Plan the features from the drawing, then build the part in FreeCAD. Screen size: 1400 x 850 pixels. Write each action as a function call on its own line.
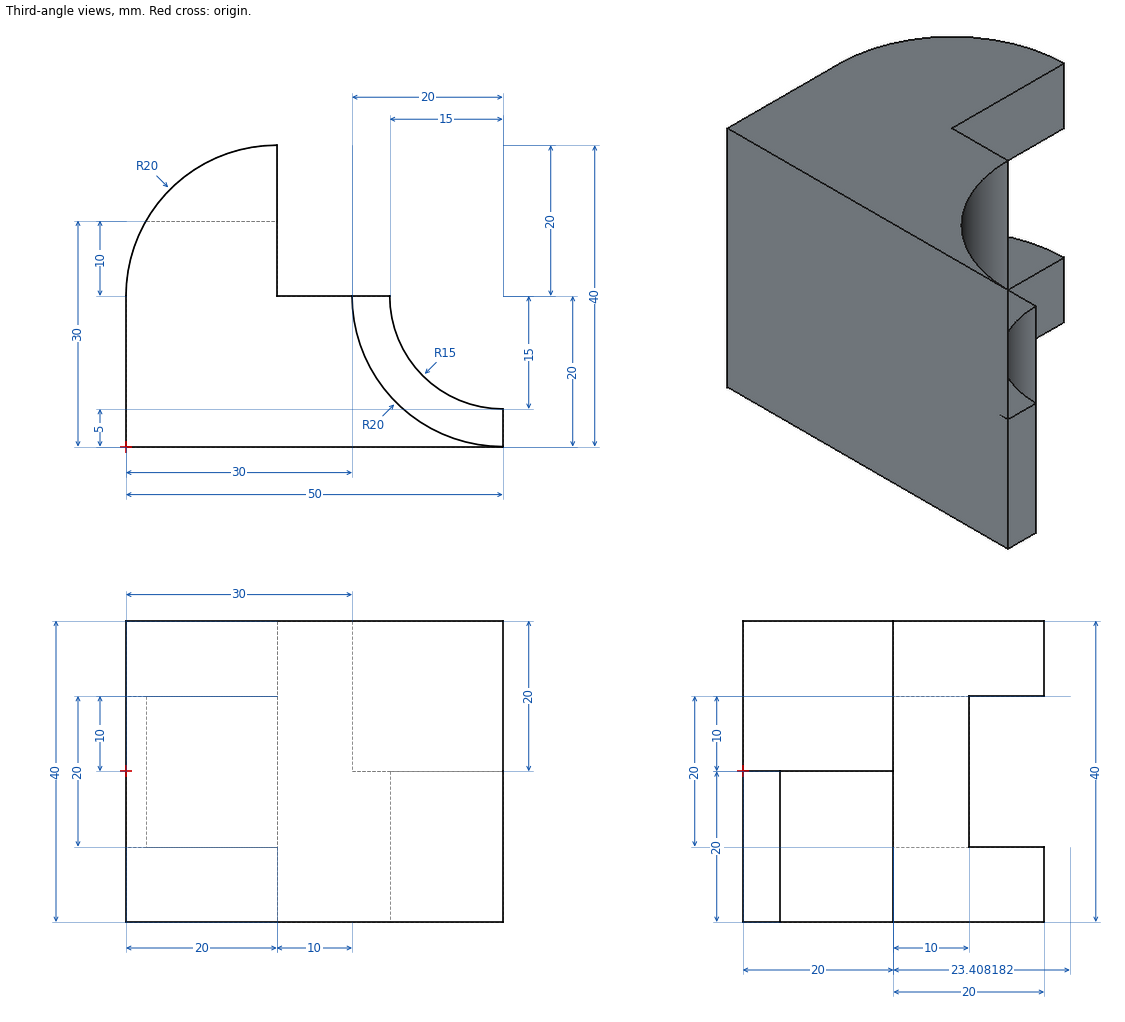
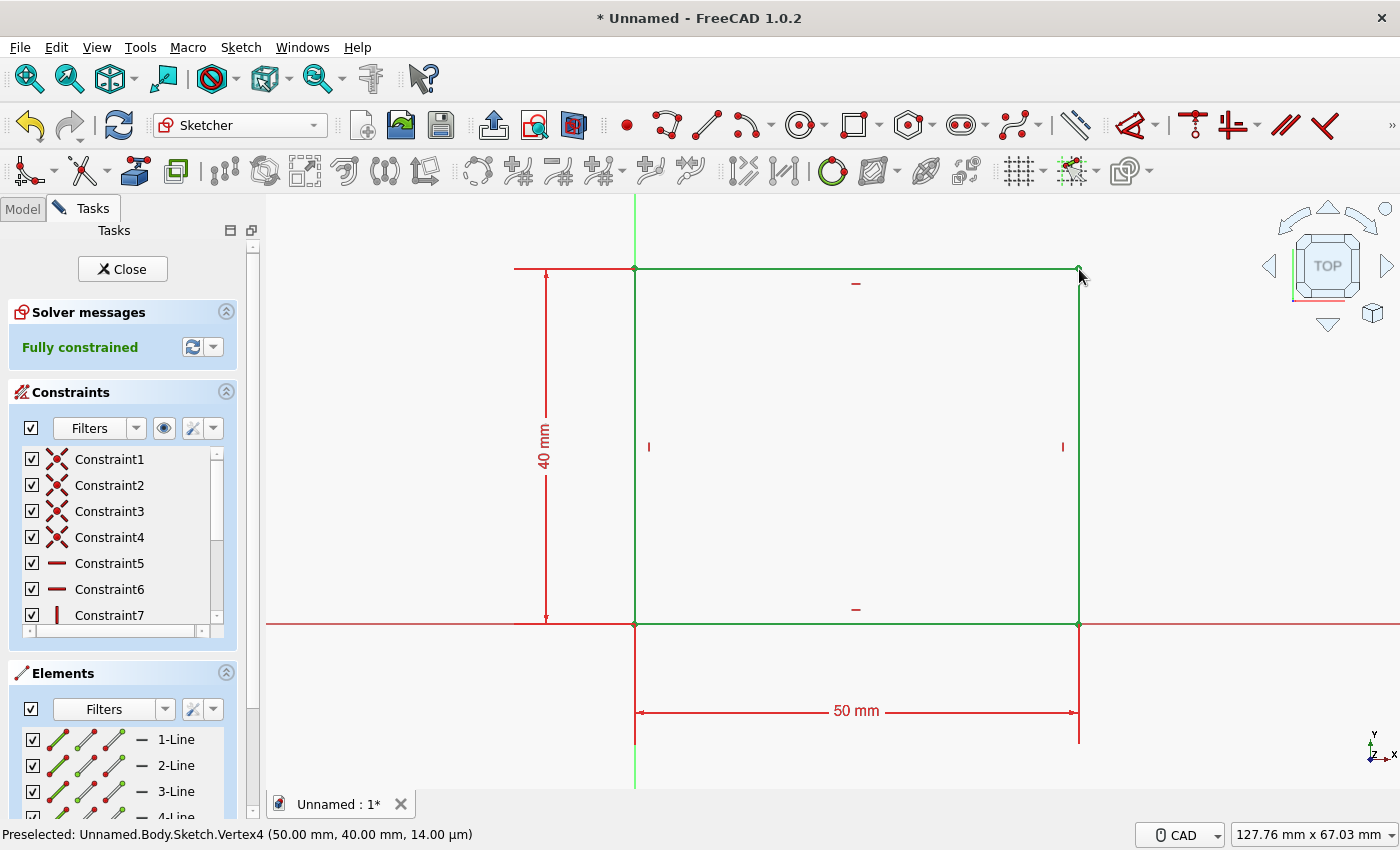
click(123, 269)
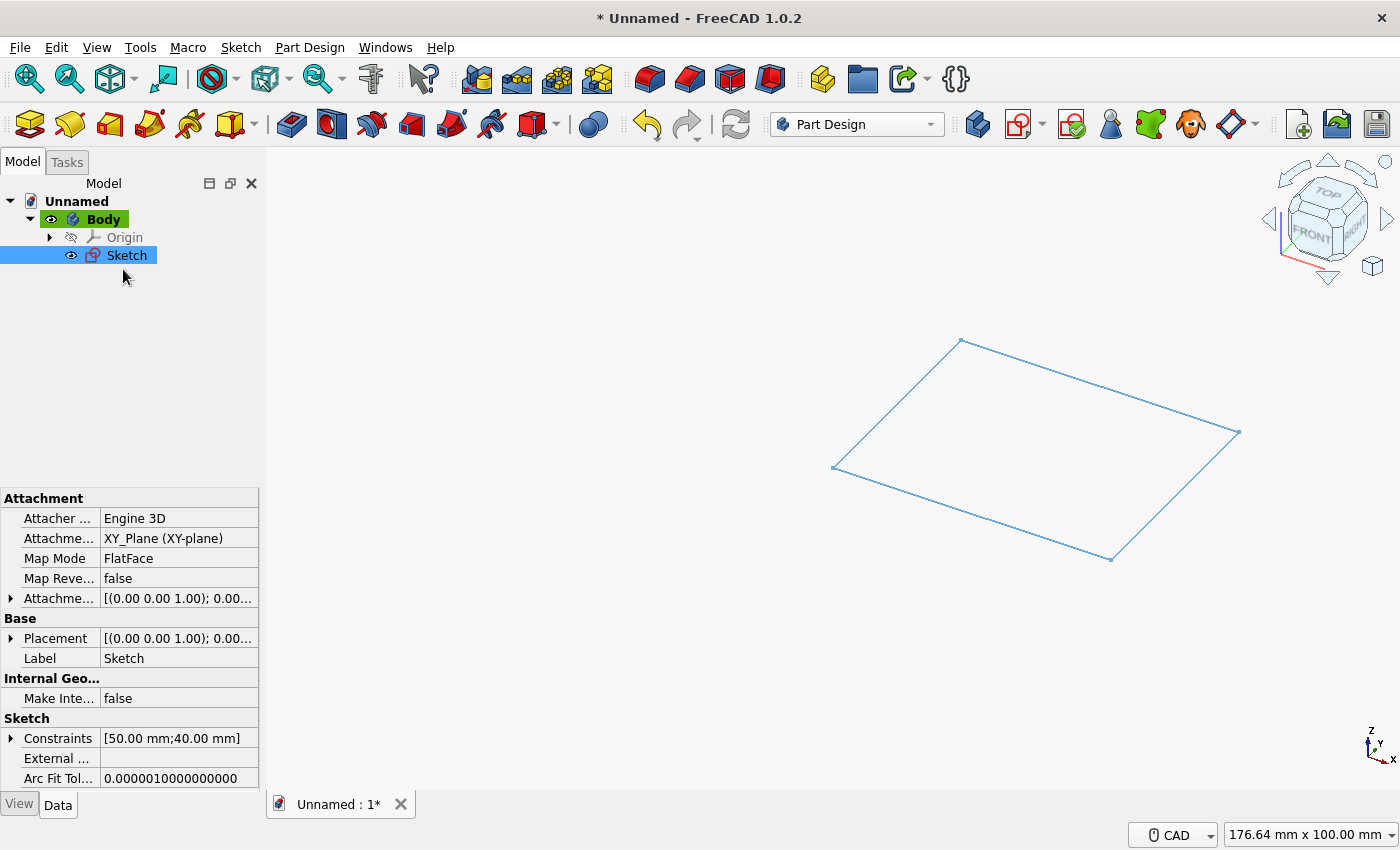
click(30, 124)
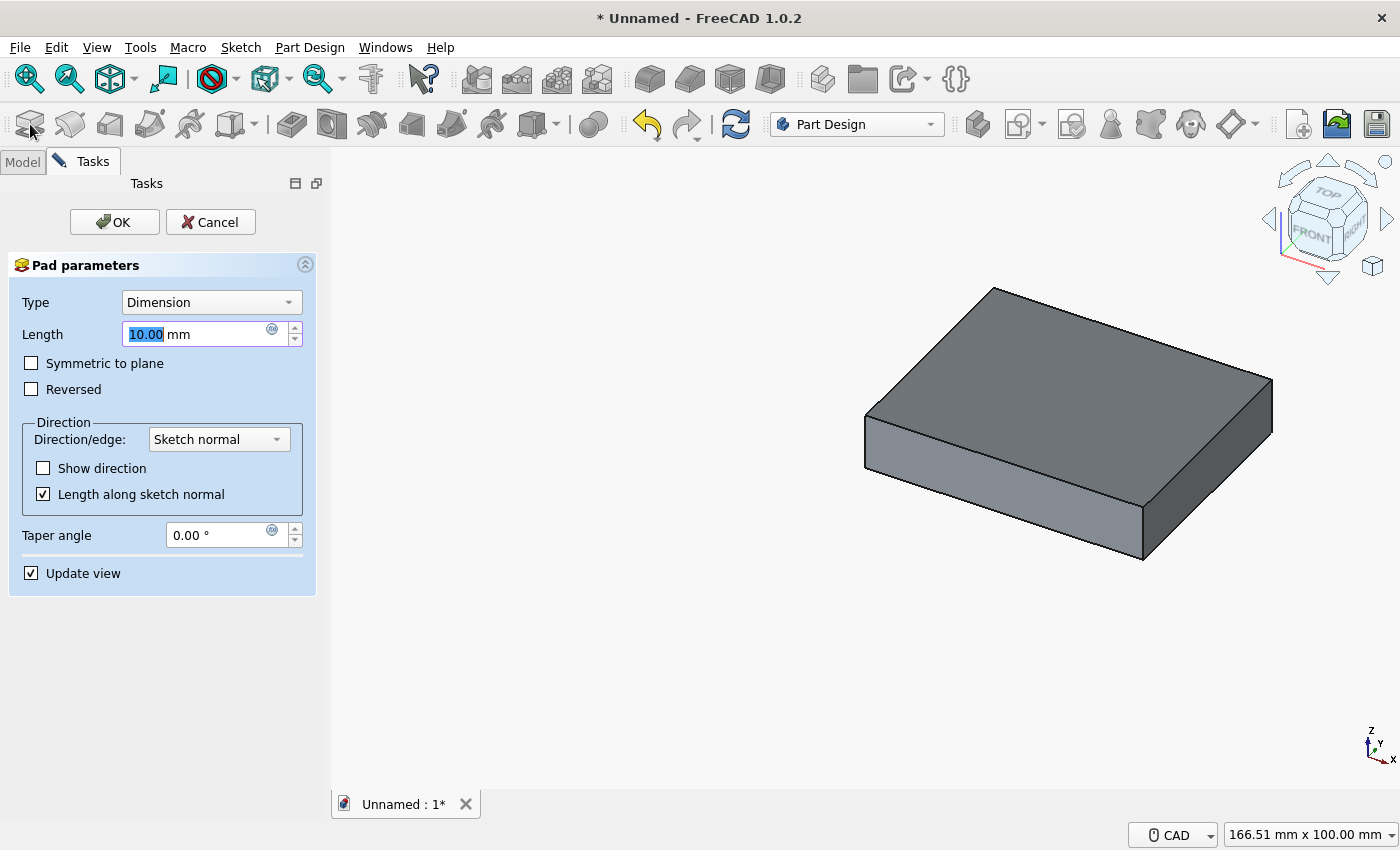
text(40)
key(Tab)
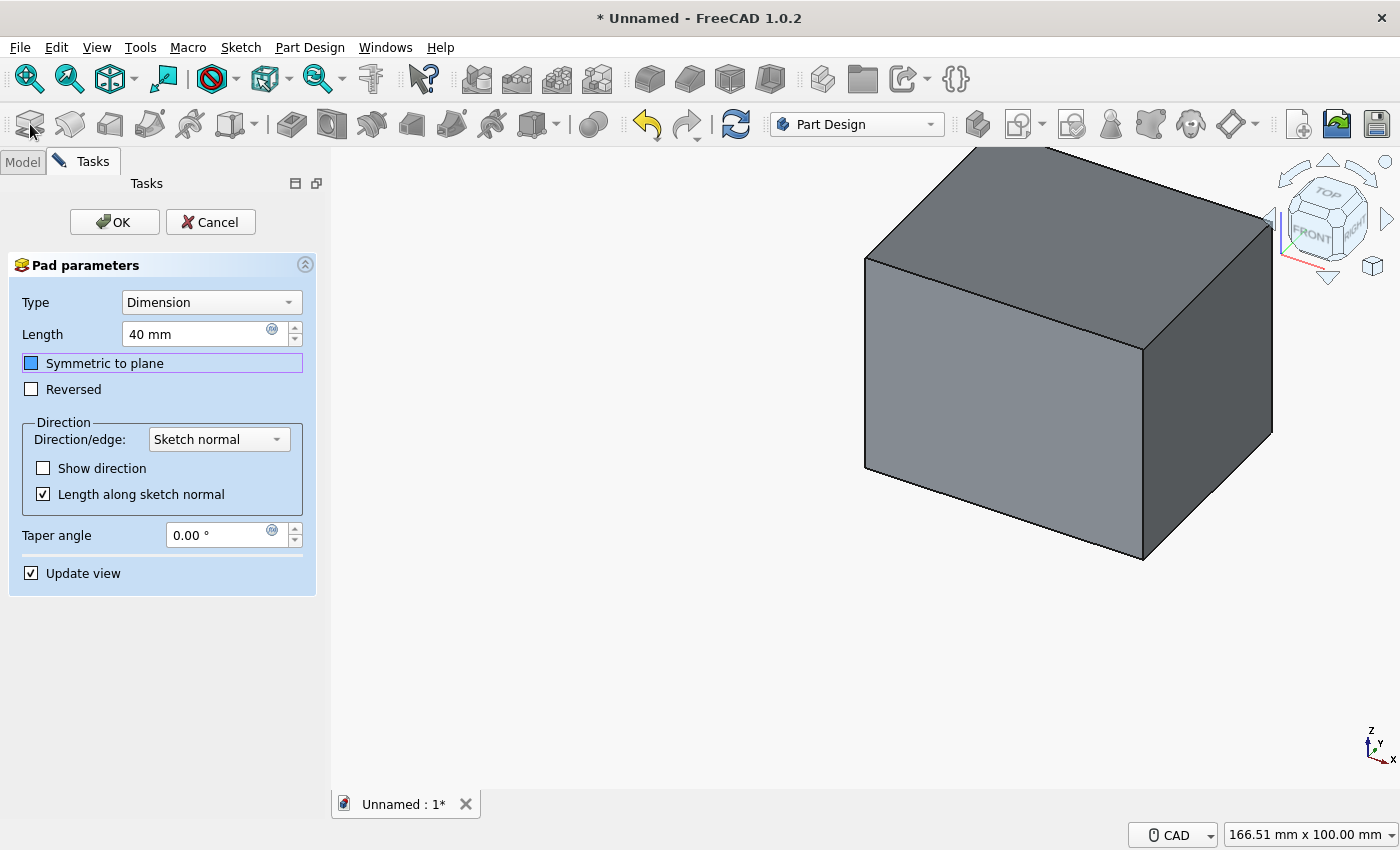
click(30, 363)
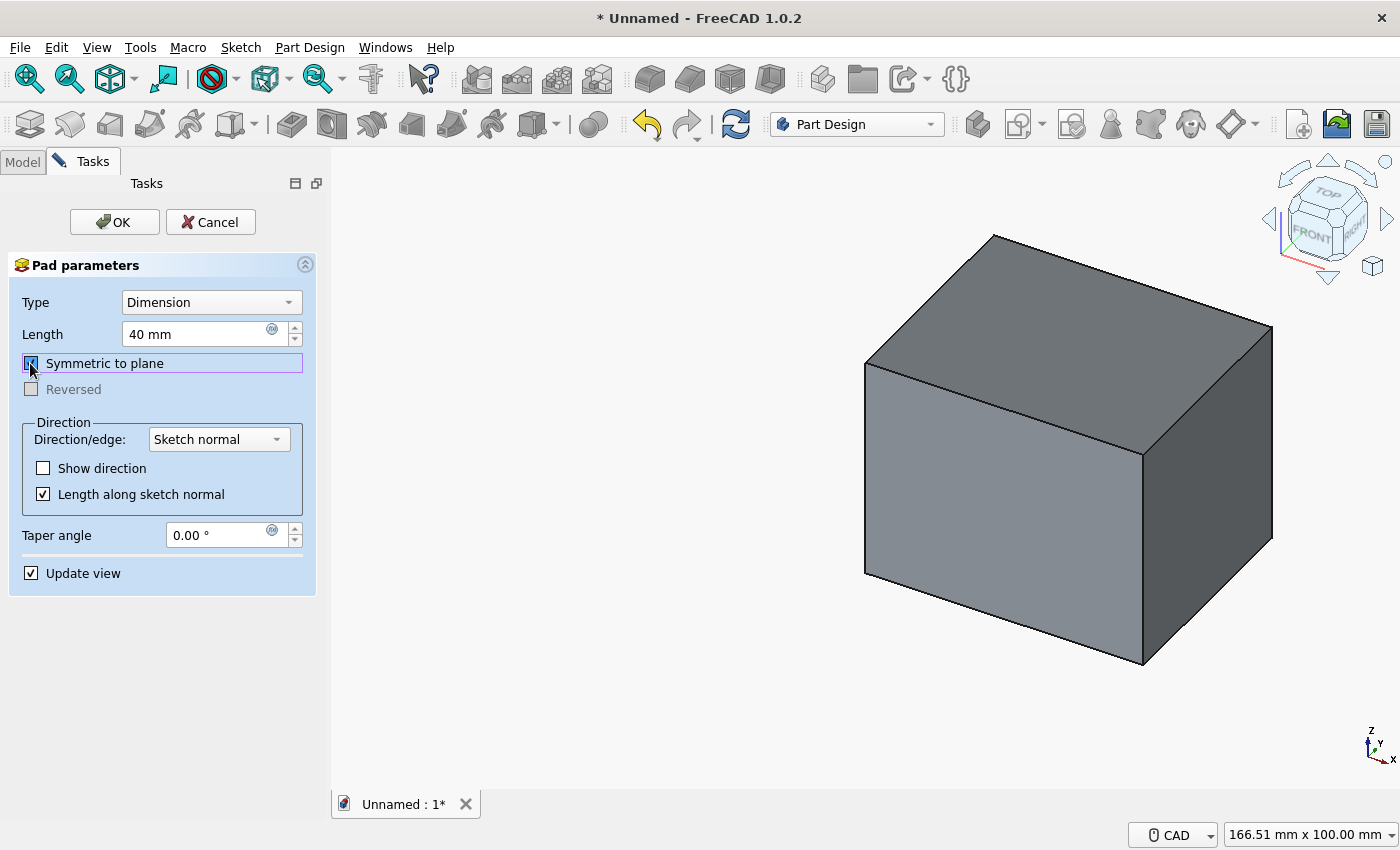
click(115, 222)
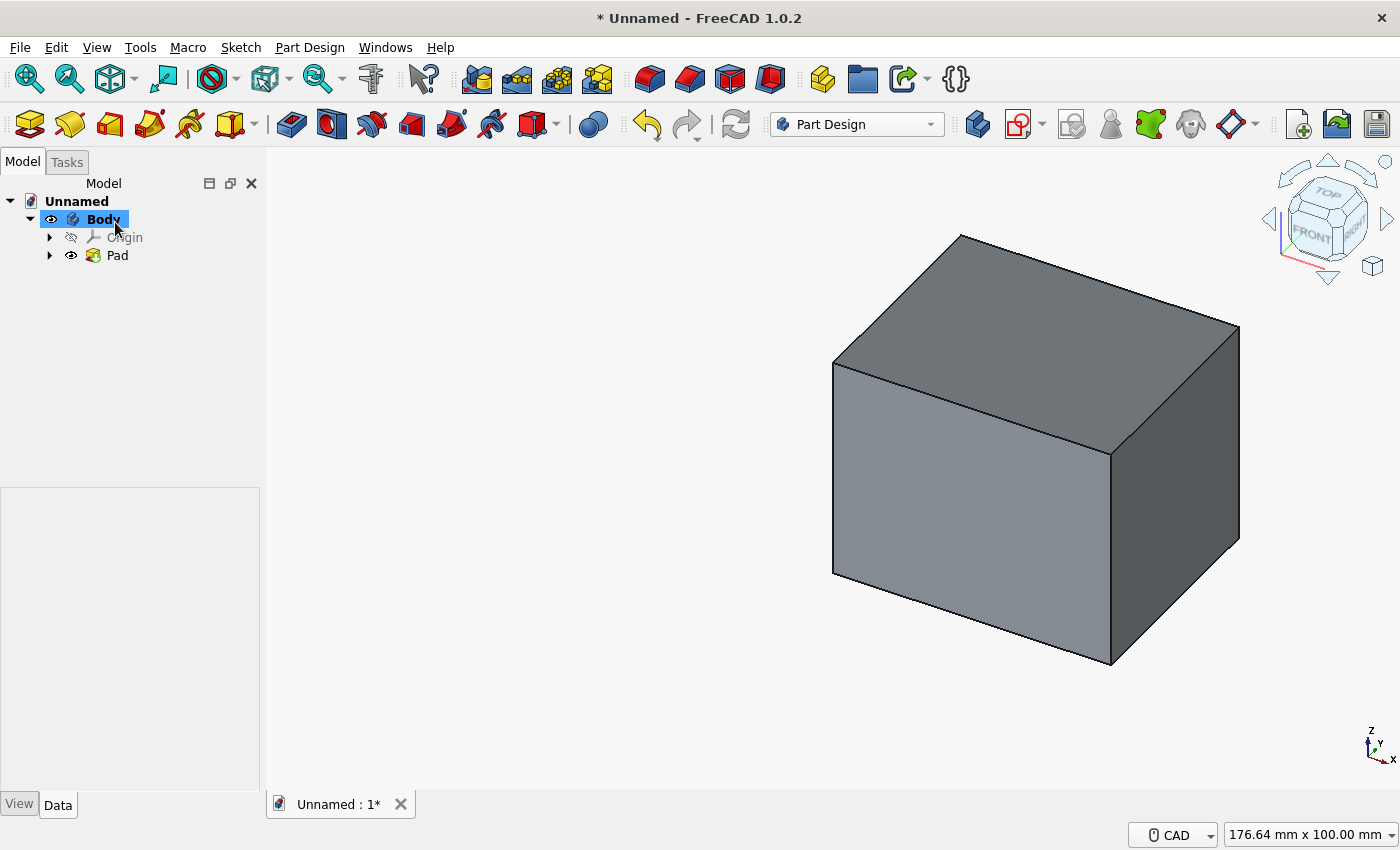
click(1036, 344)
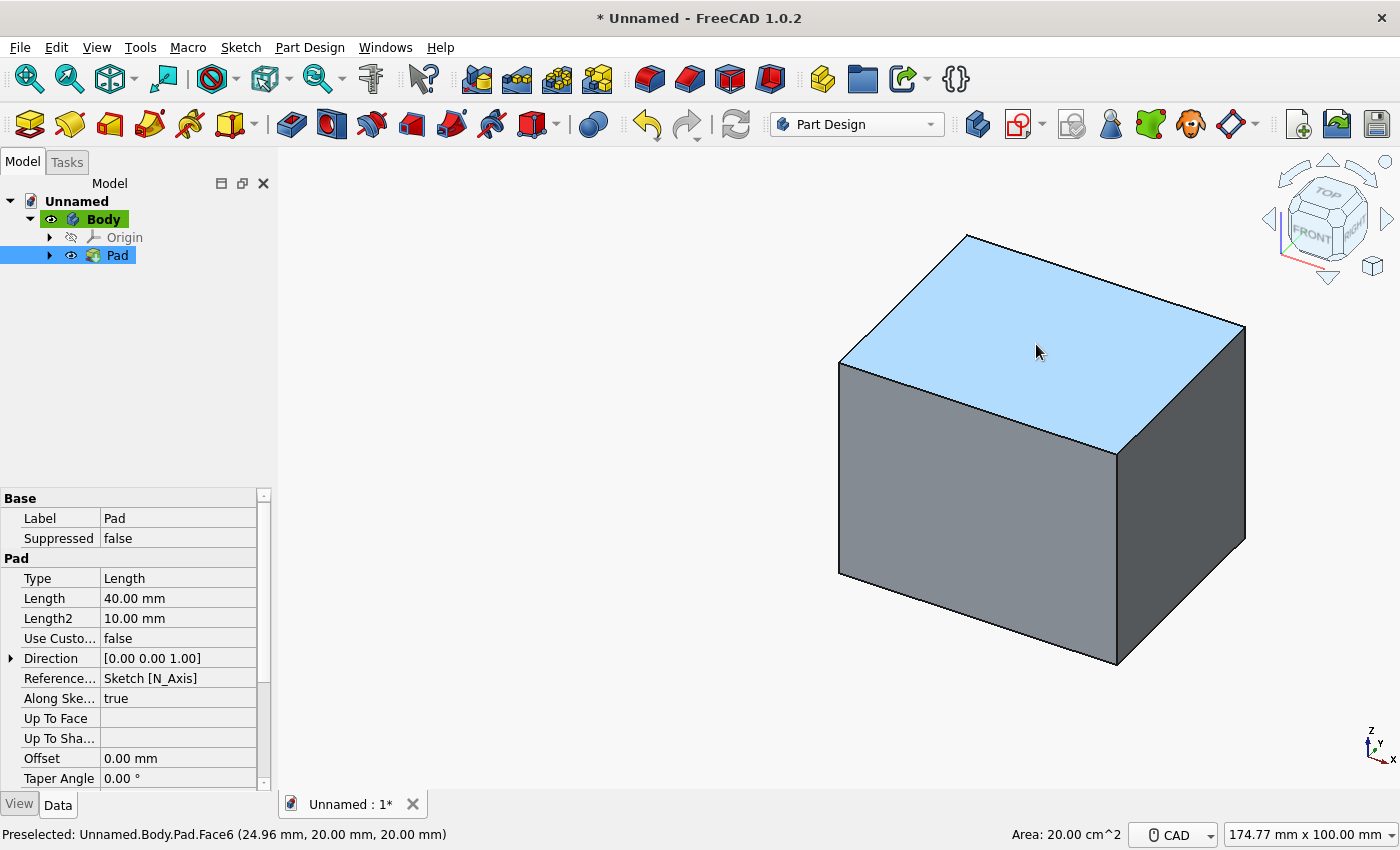
click(1018, 124)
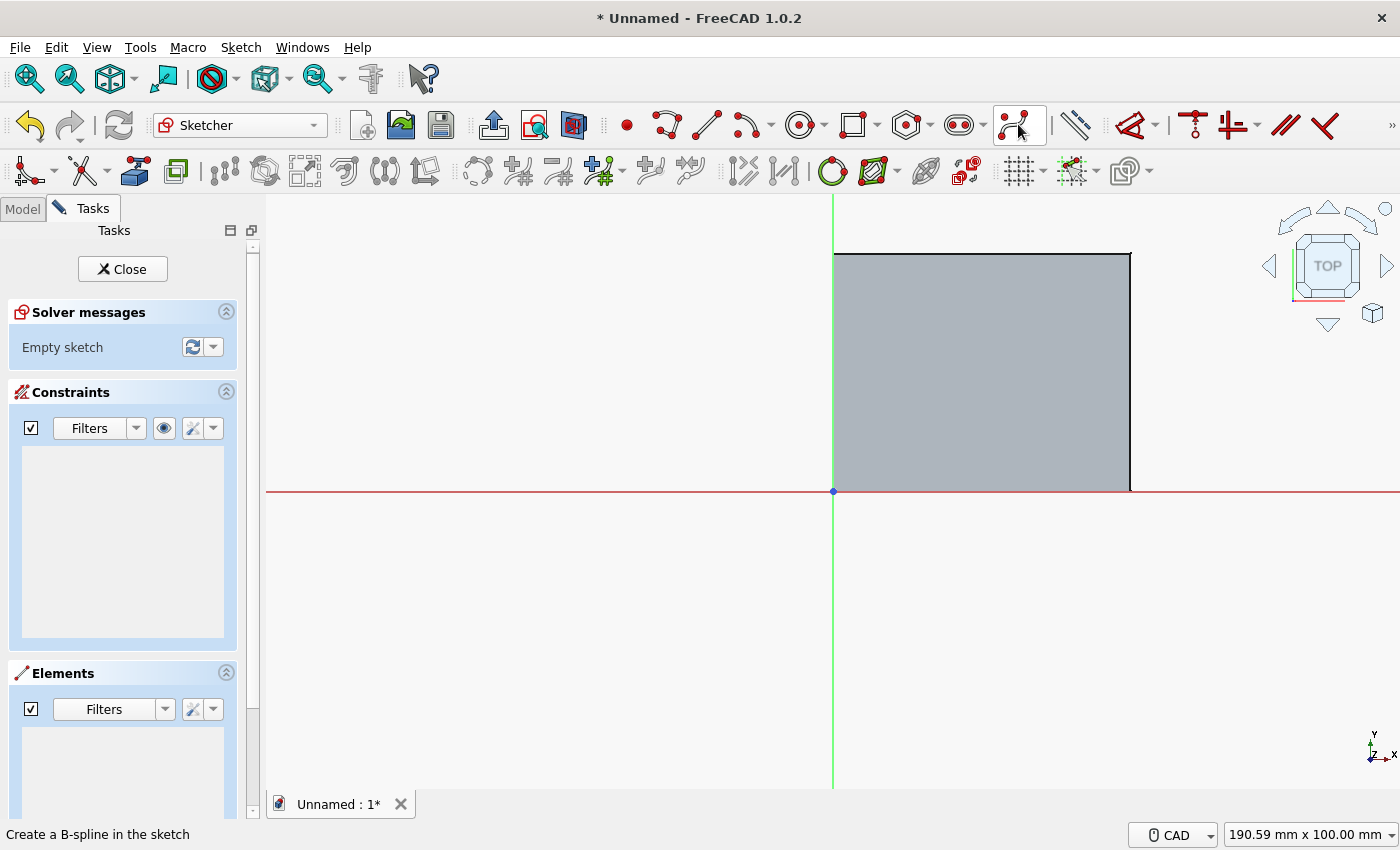
scroll(1203, 236, up, 6)